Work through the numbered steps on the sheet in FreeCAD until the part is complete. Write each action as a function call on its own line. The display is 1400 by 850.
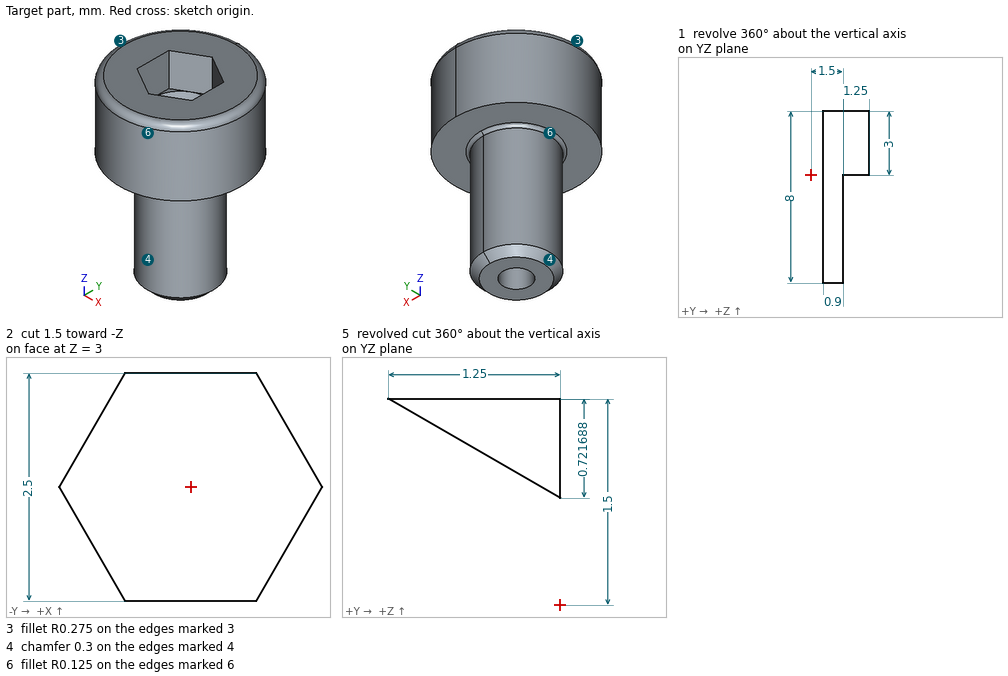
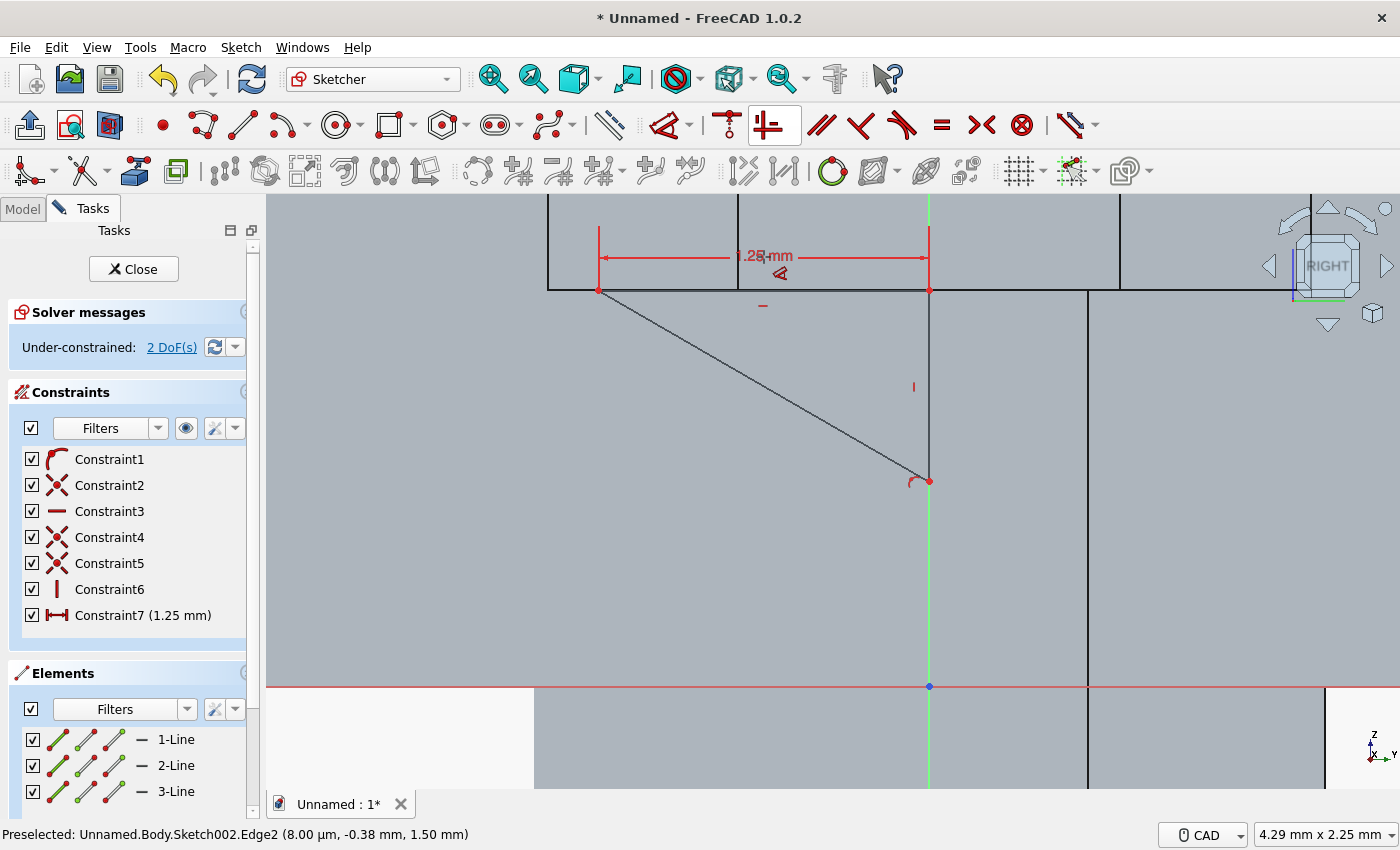
click(929, 291)
click(963, 489)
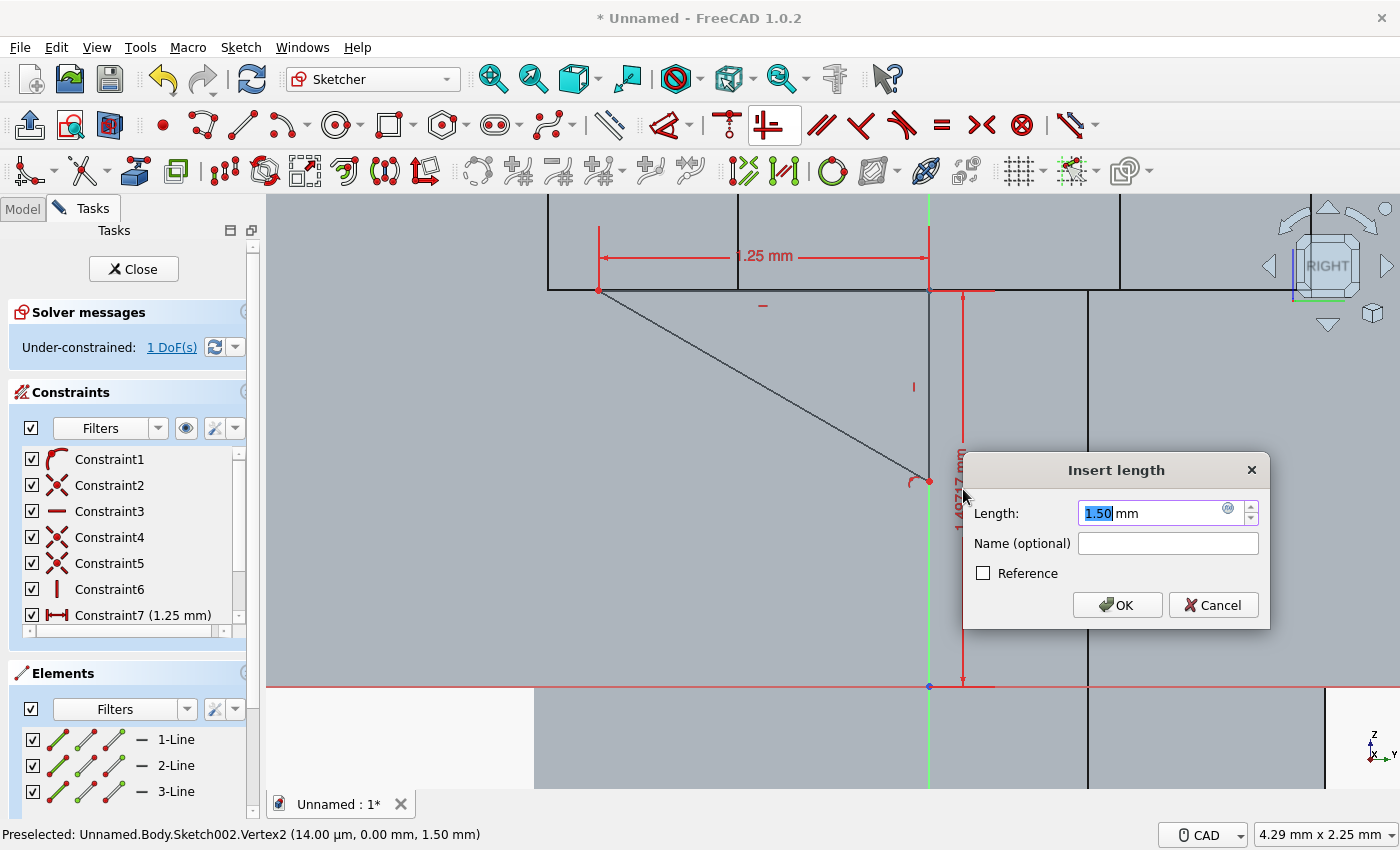
text(1.5)
key(Return)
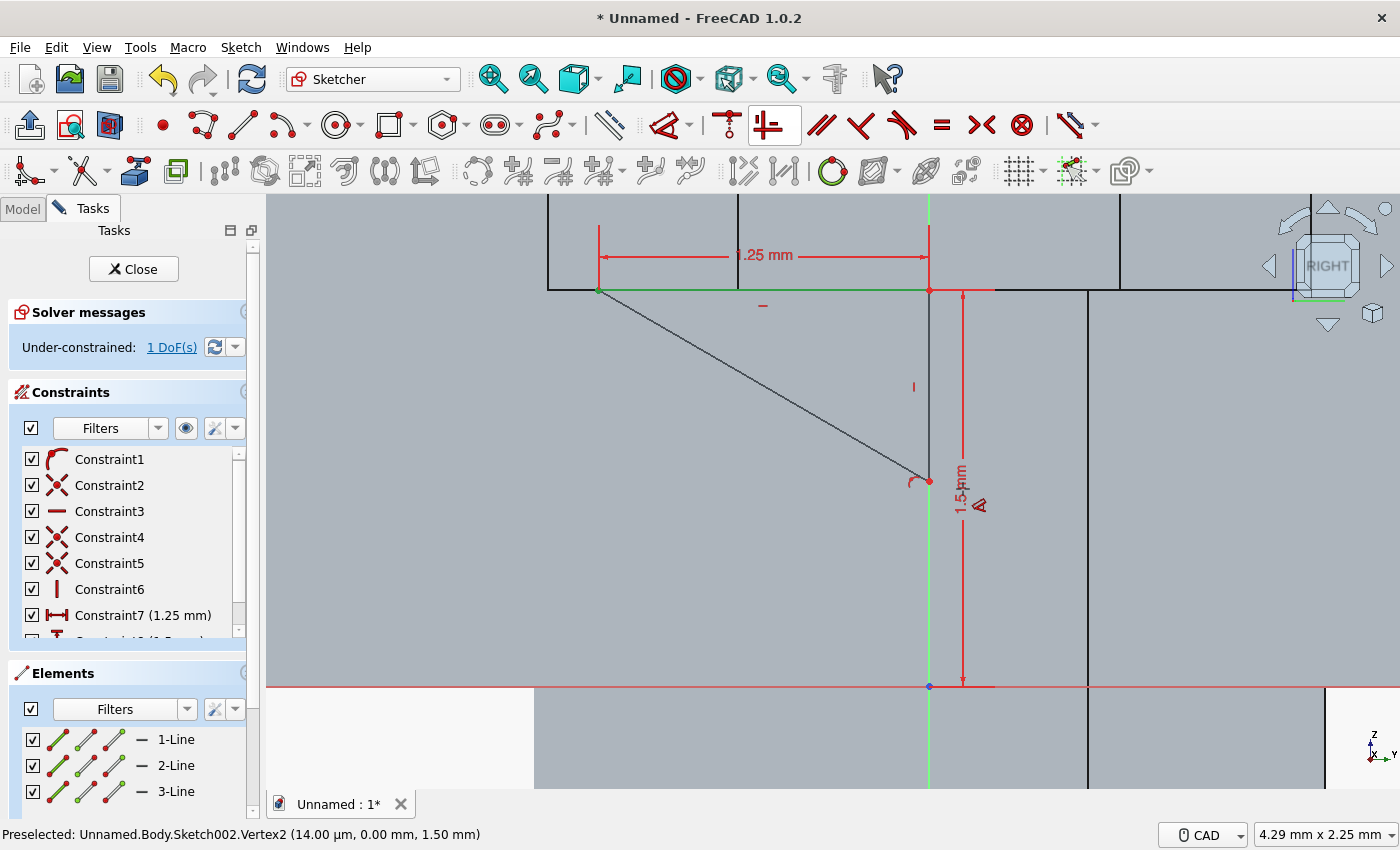
click(929, 424)
click(963, 386)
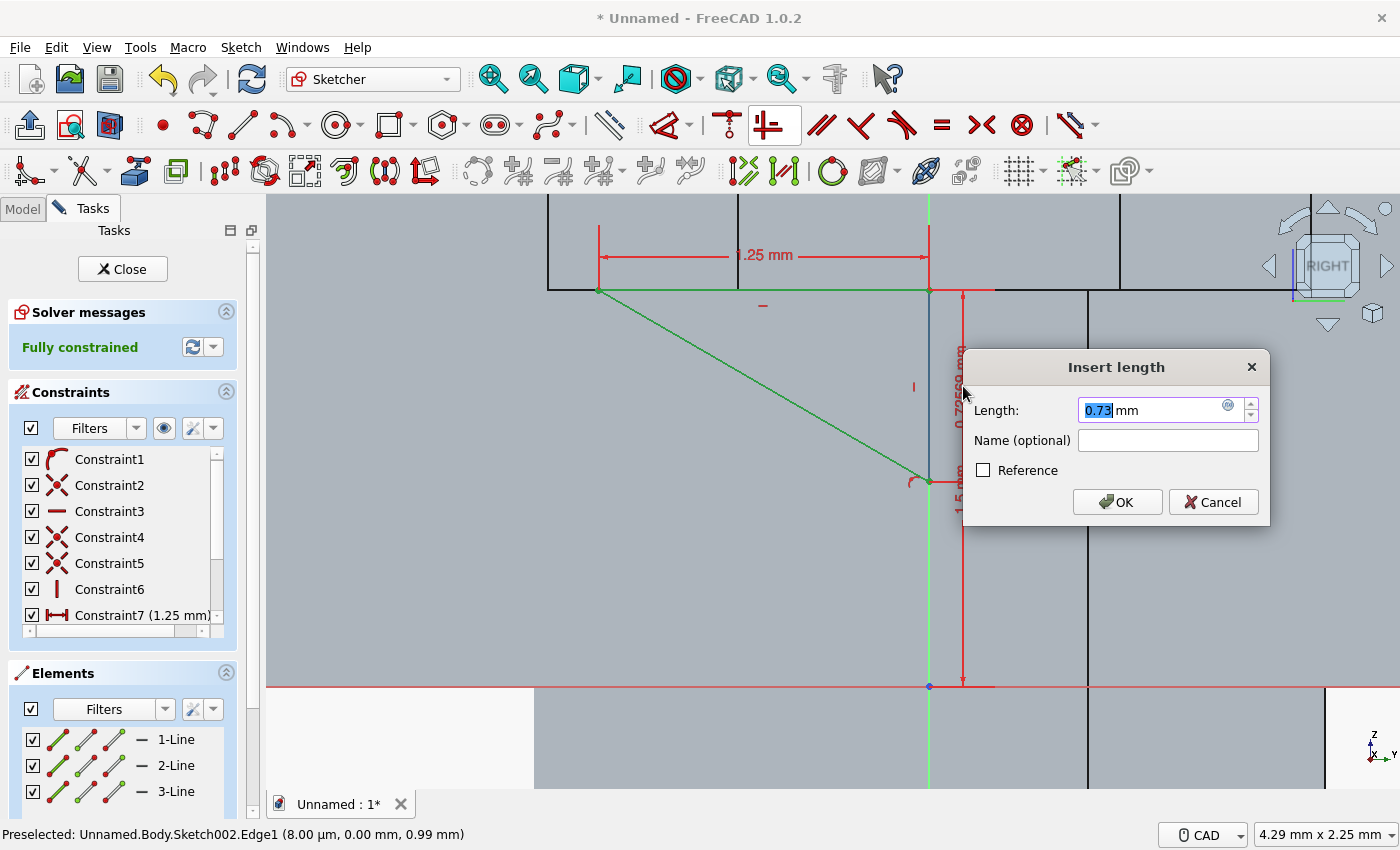
text(0.721688)
key(Return)
key(Escape)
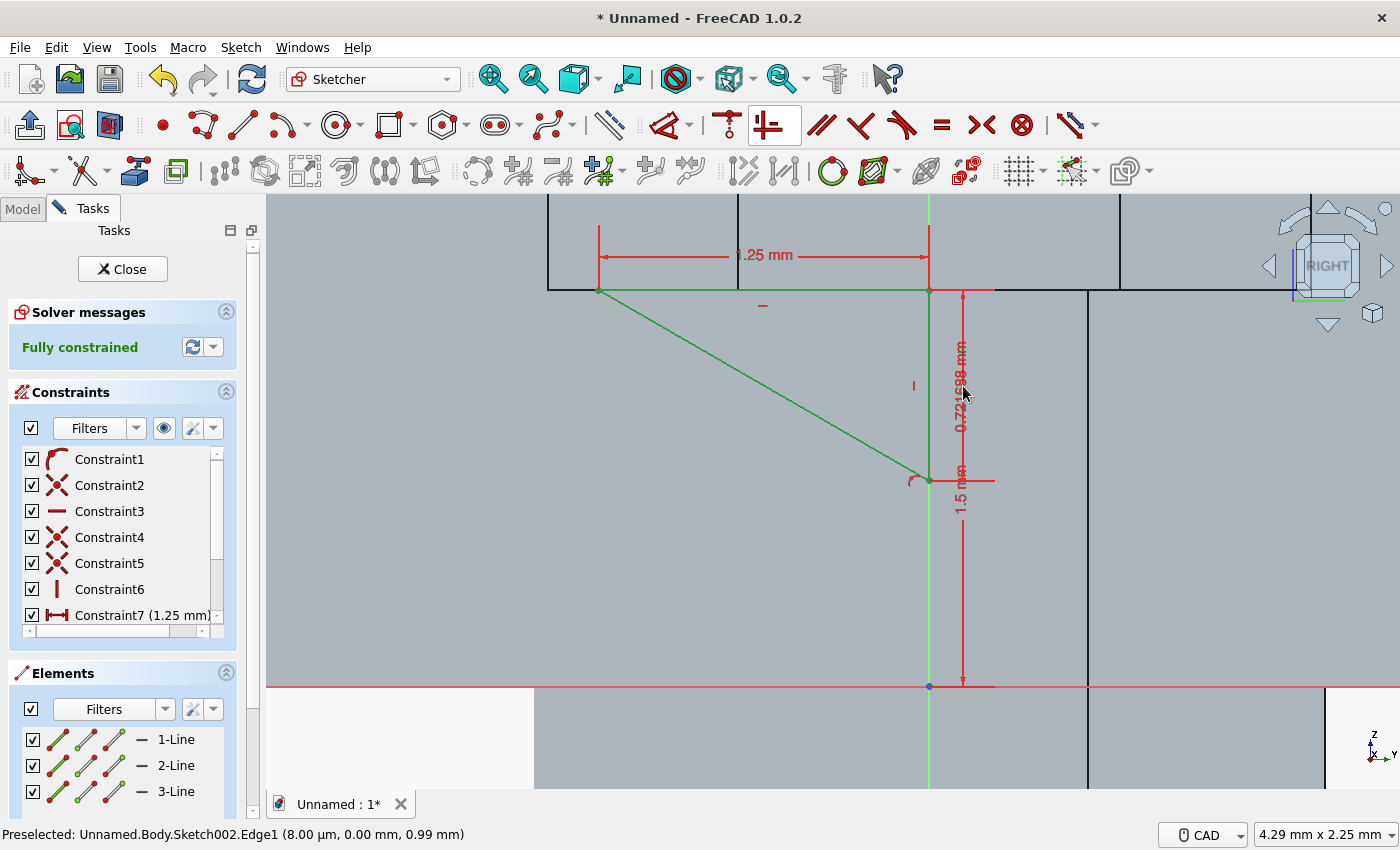
click(123, 269)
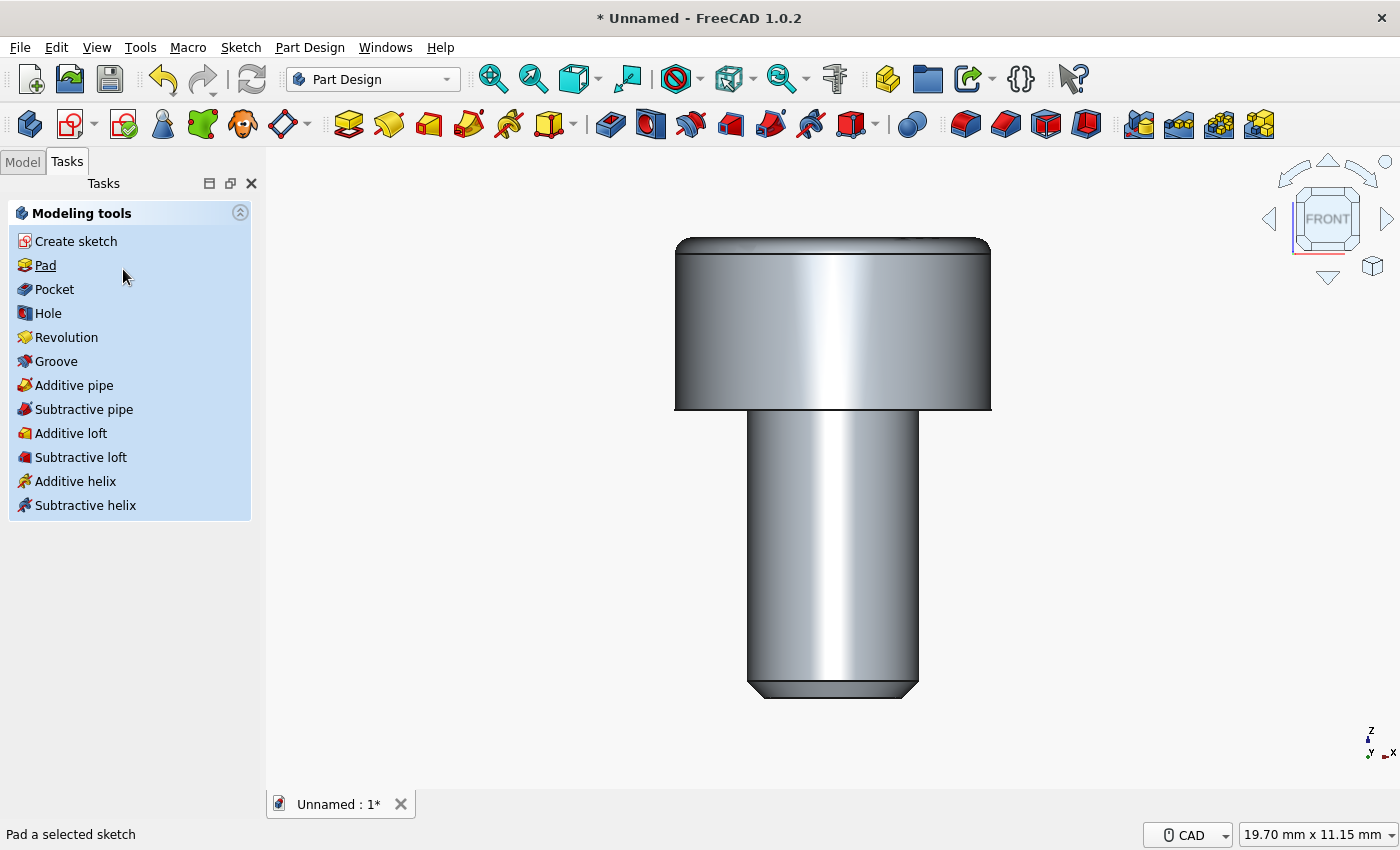
click(692, 124)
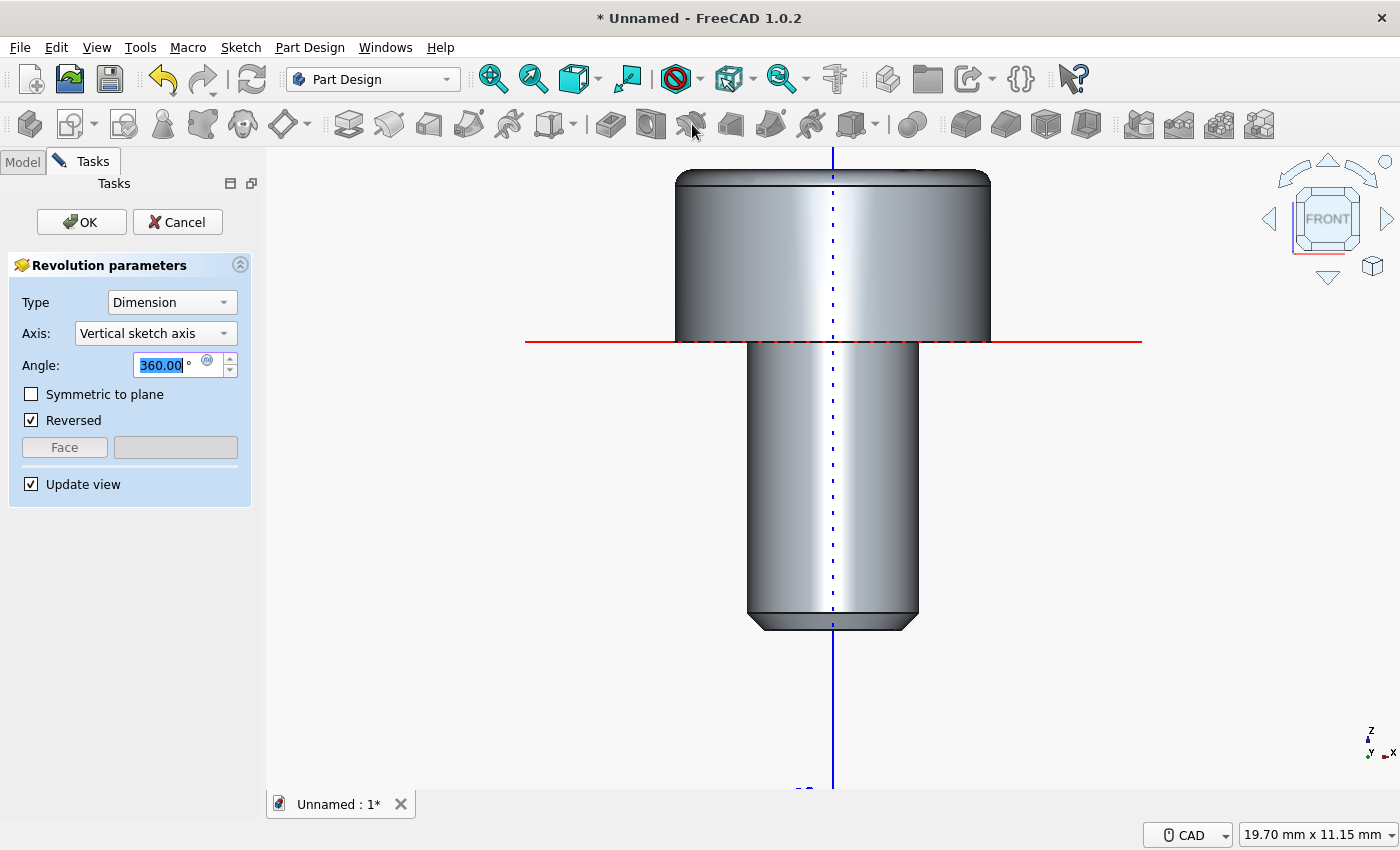
click(82, 222)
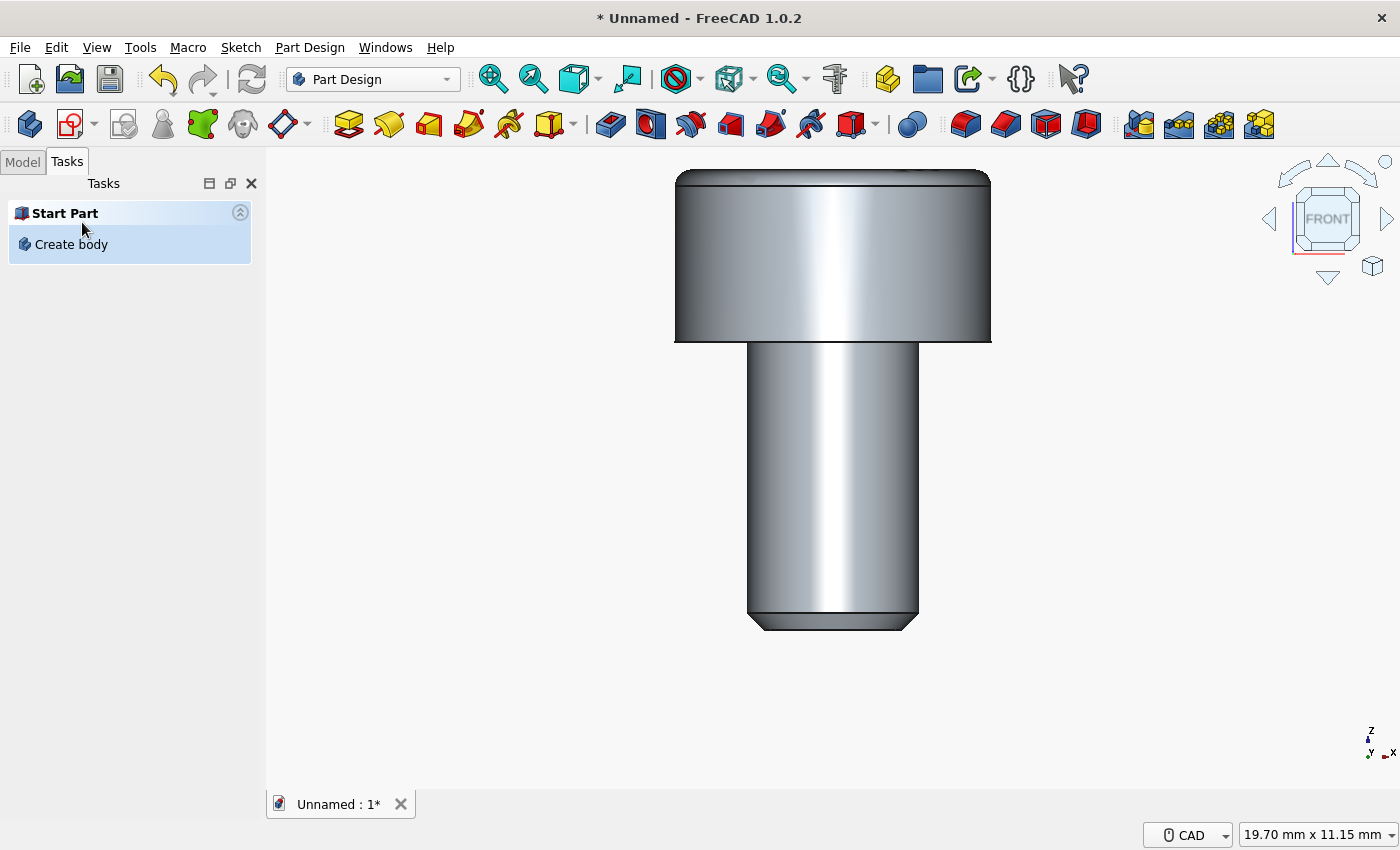
key(0)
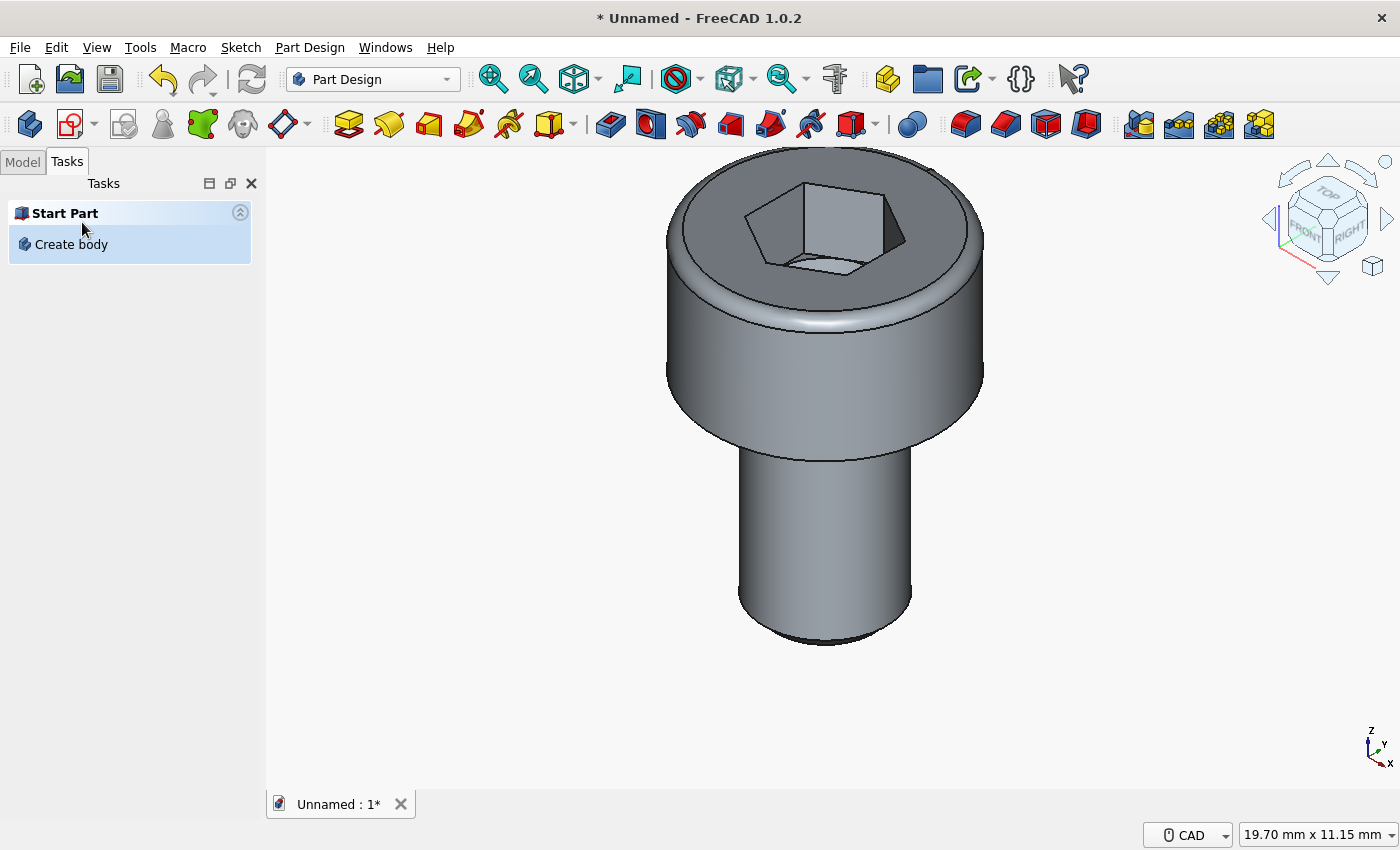
click(494, 80)